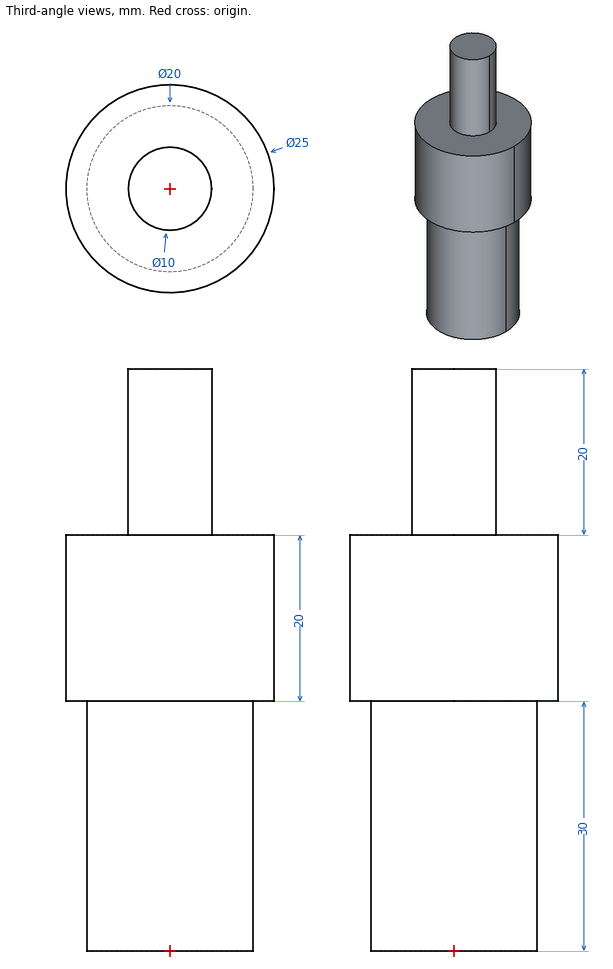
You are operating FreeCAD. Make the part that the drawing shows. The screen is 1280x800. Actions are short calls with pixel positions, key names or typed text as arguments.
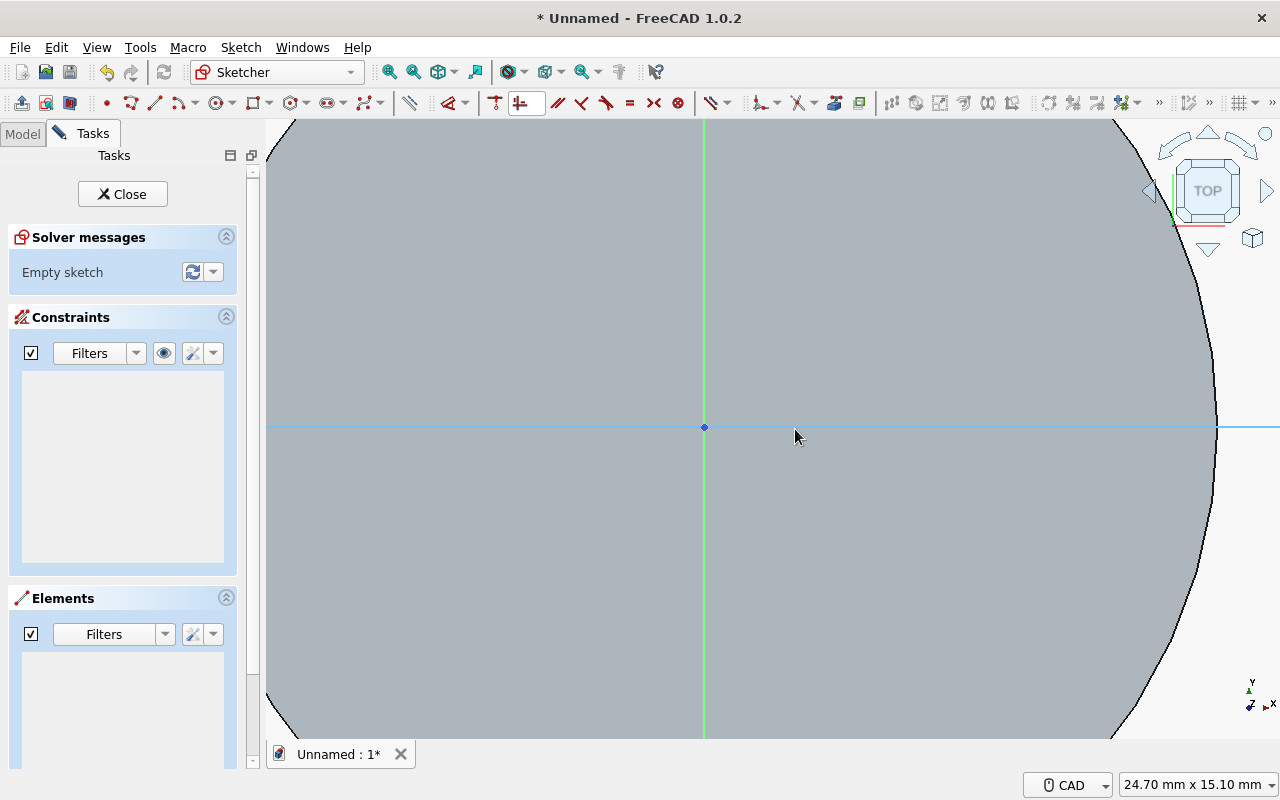
click(216, 104)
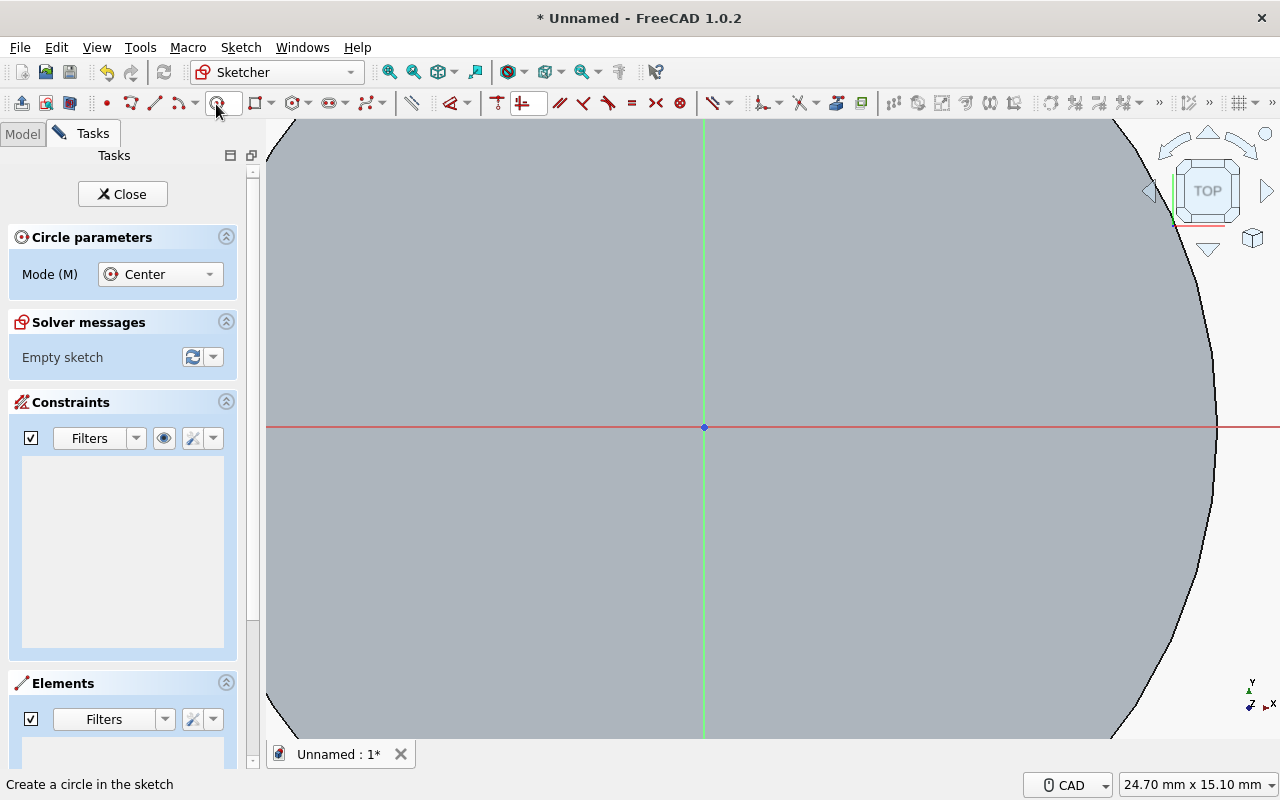
click(704, 427)
click(849, 282)
key(Escape)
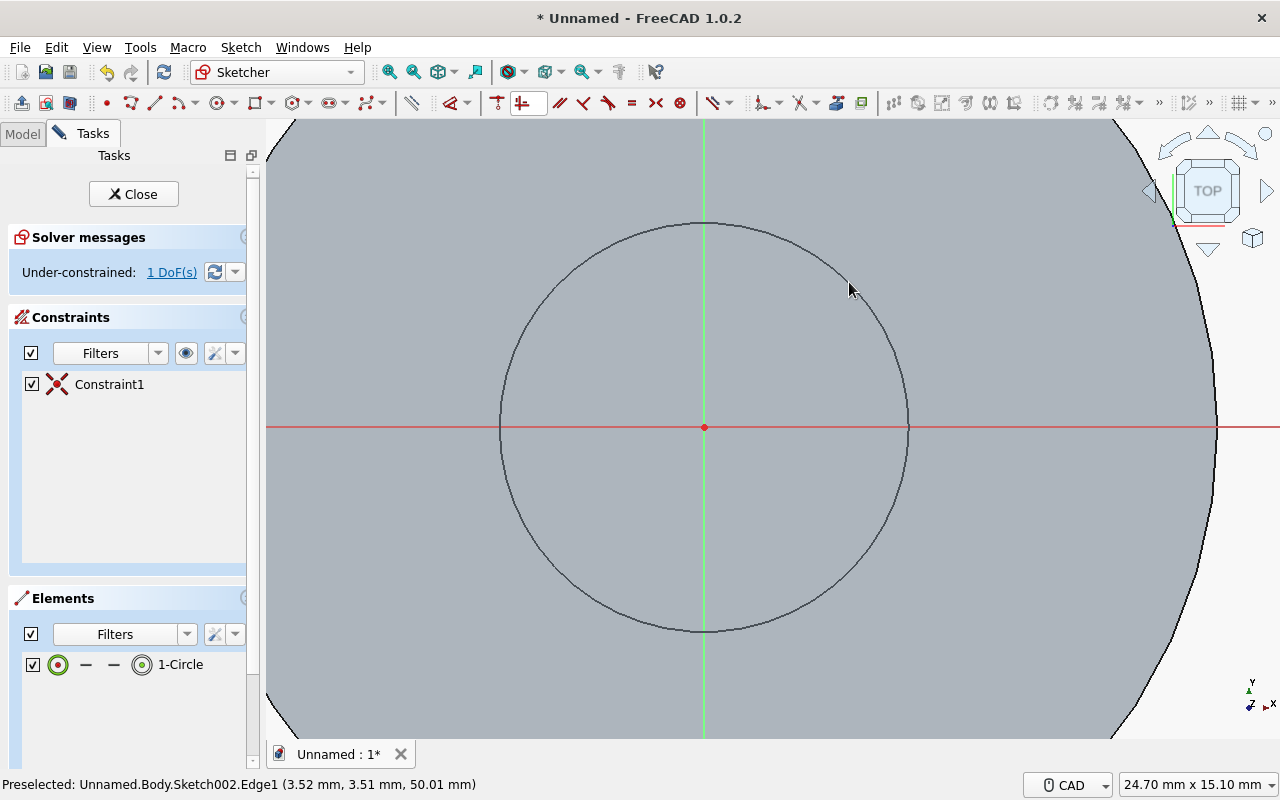
key(d)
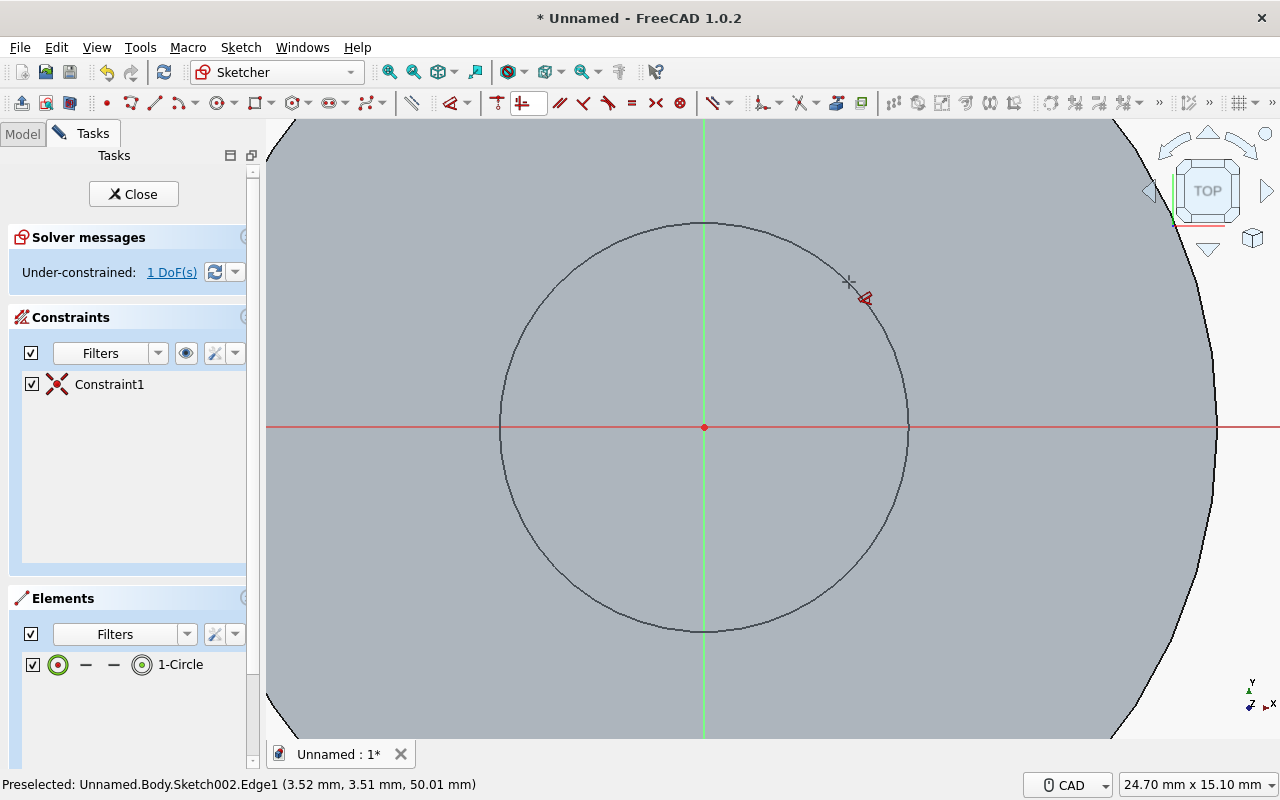
click(848, 282)
click(870, 259)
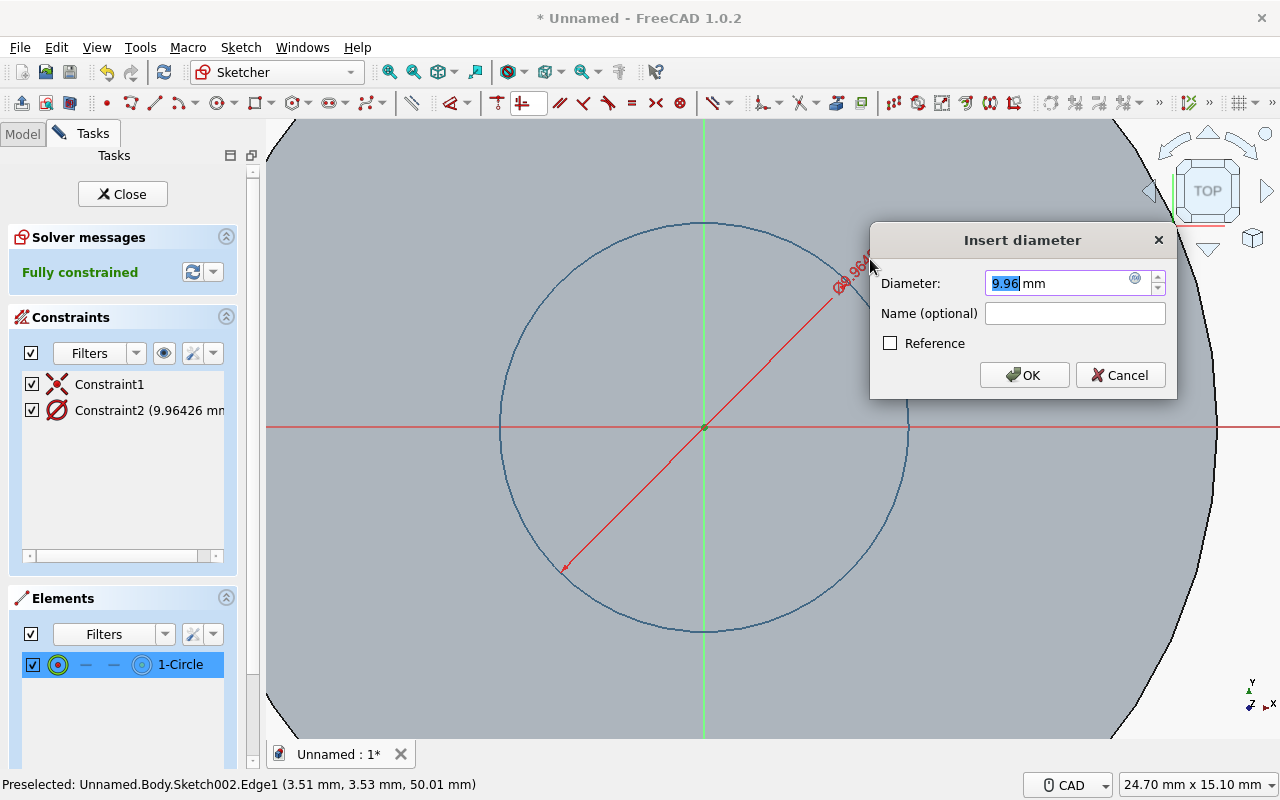
text(10)
key(Return)
key(Escape)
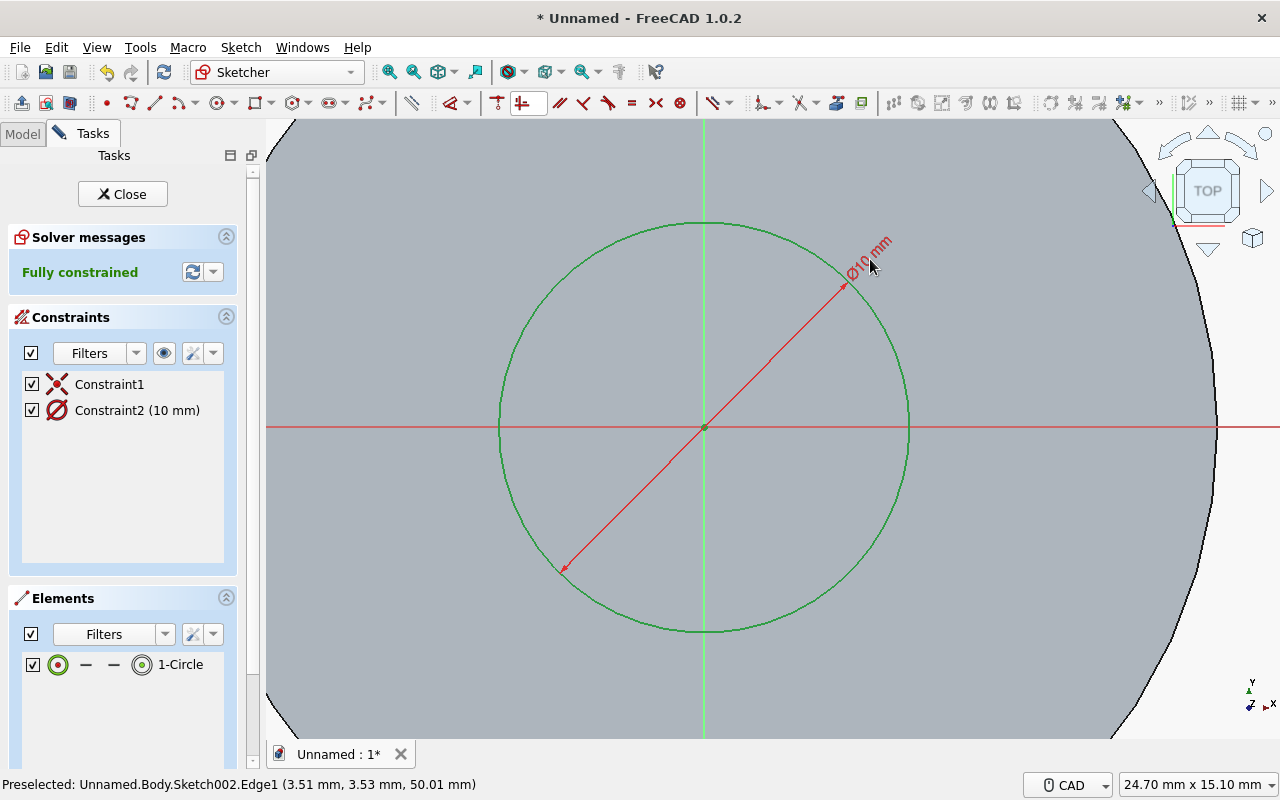
click(123, 194)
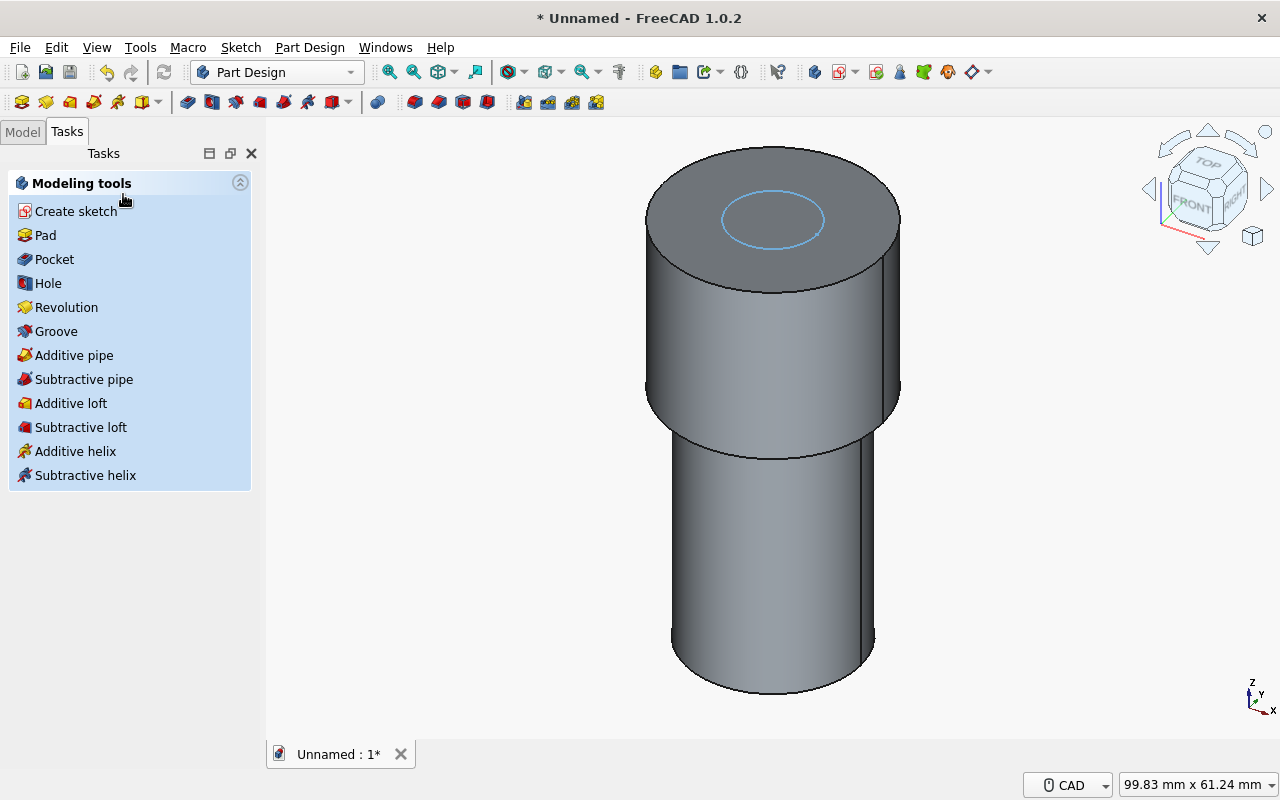
click(22, 102)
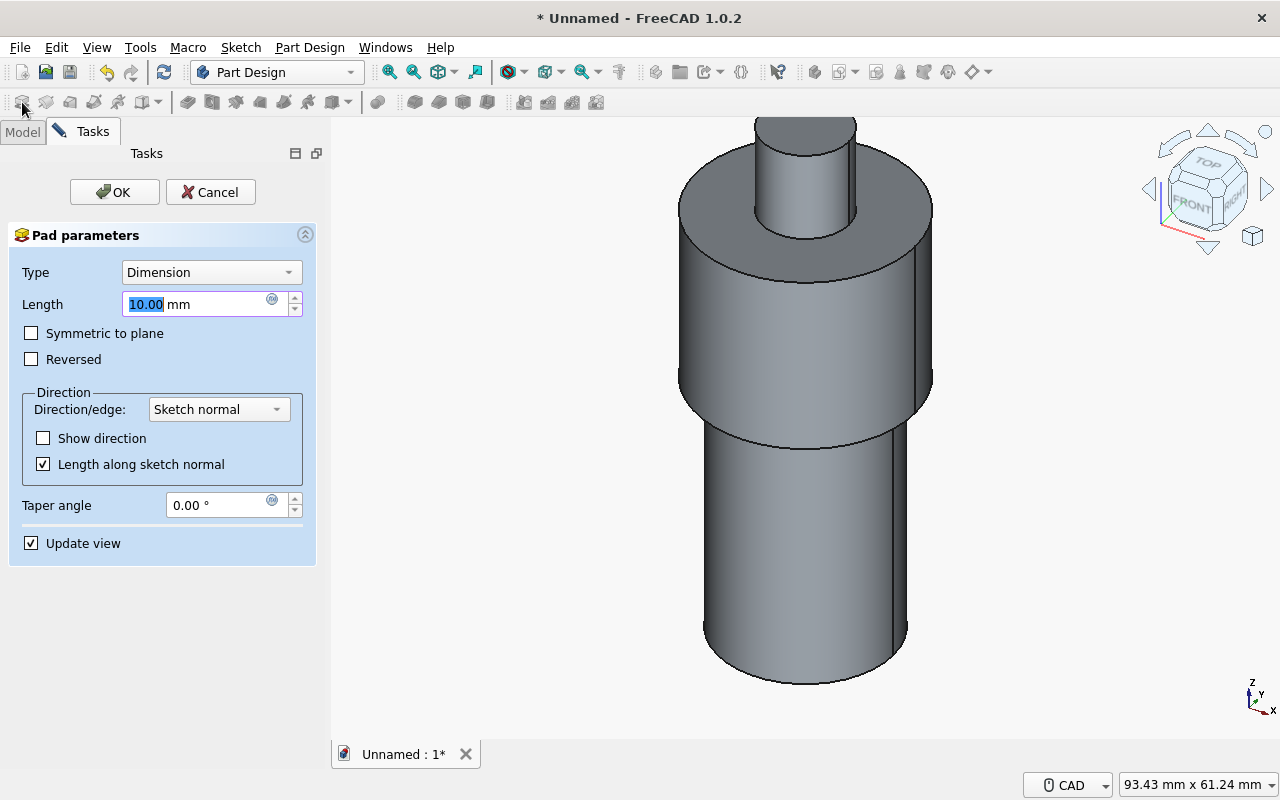
text(20)
key(Tab)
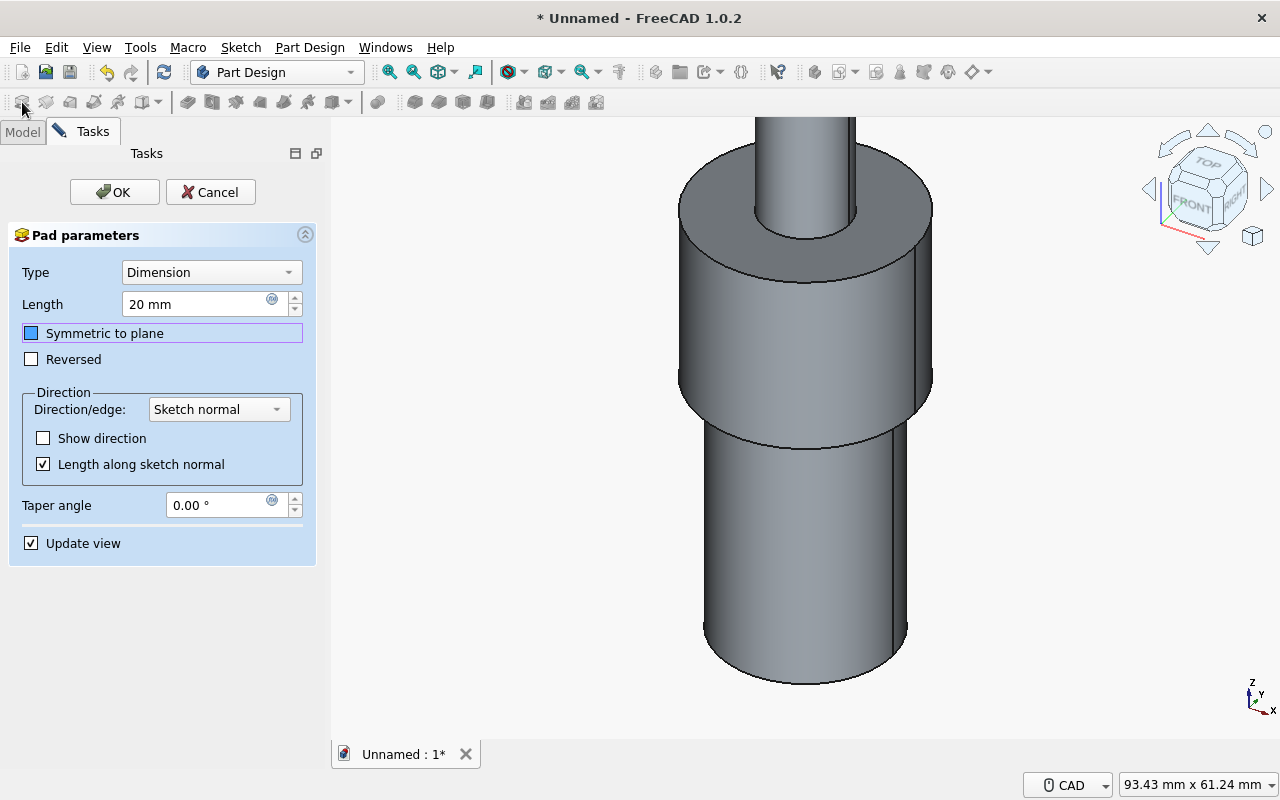
click(115, 192)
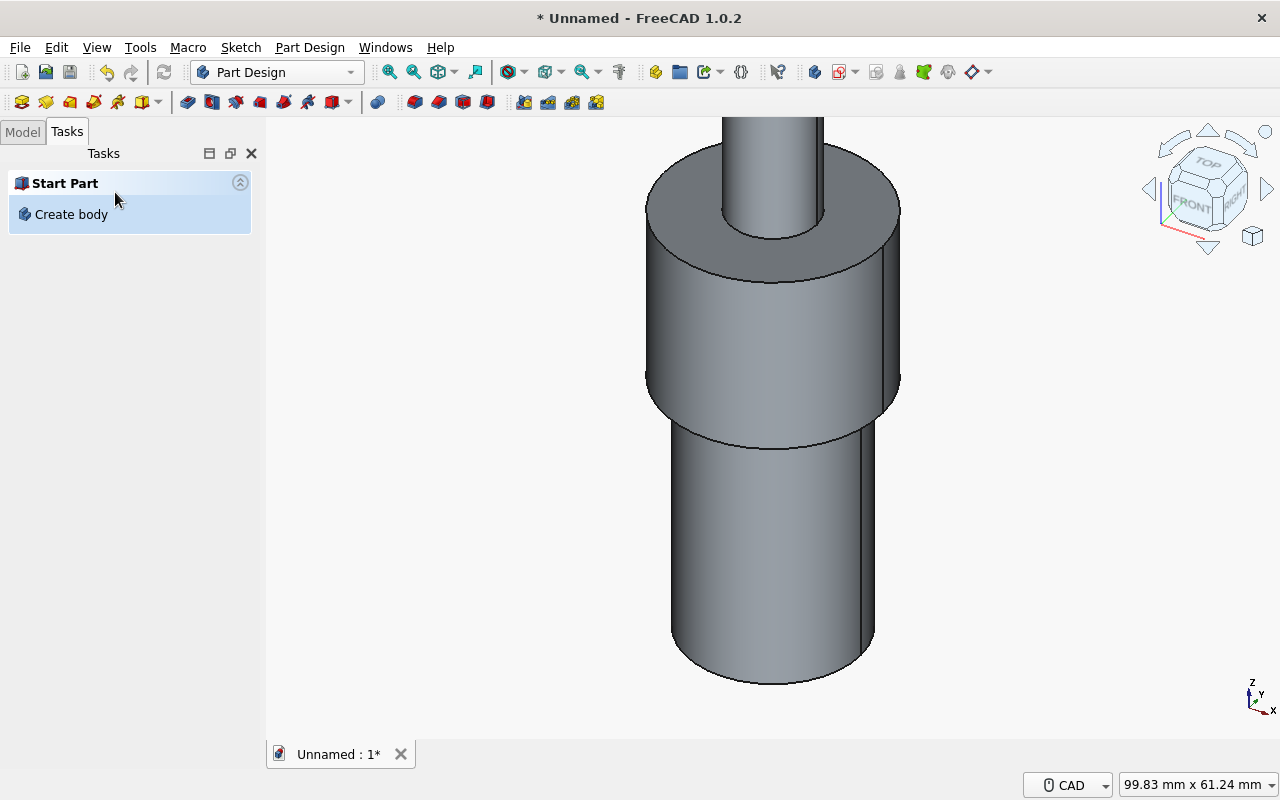
key(0)